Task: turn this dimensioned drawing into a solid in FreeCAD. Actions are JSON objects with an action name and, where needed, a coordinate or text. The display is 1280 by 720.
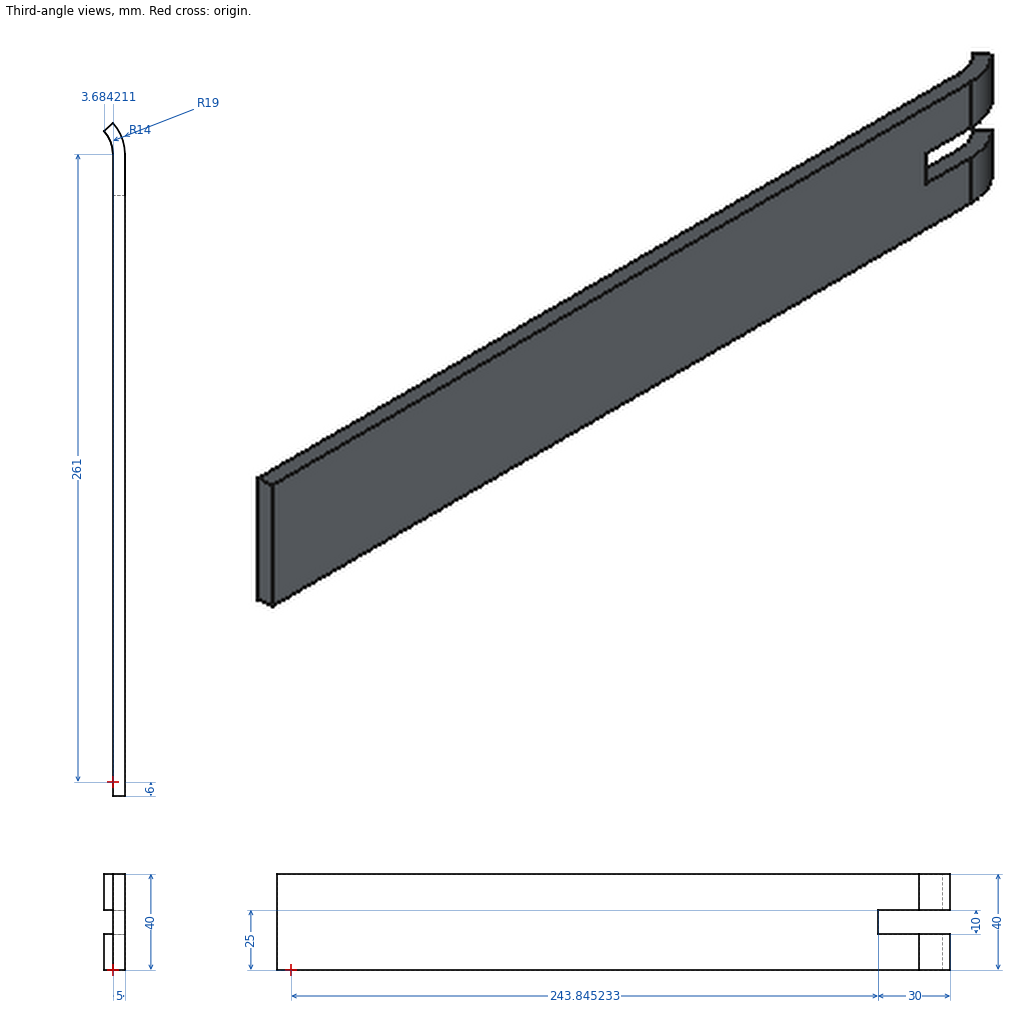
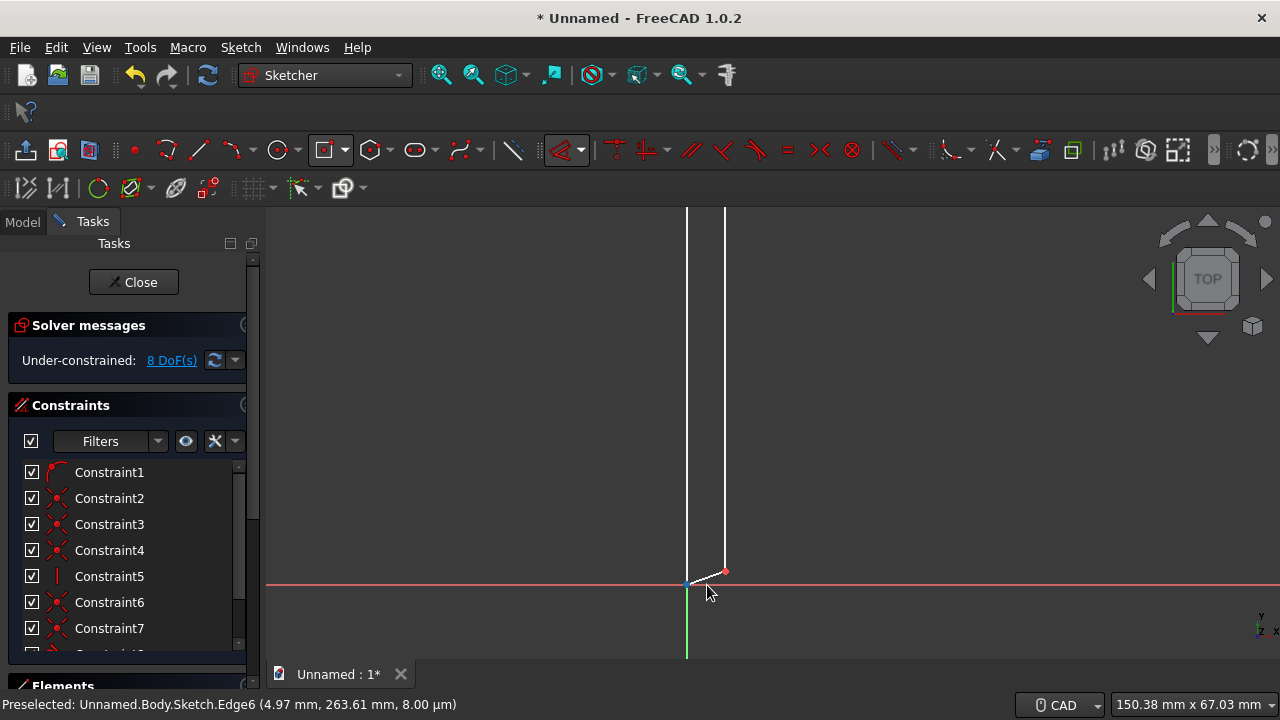
{"action": "left_click", "coordinate": [702, 579]}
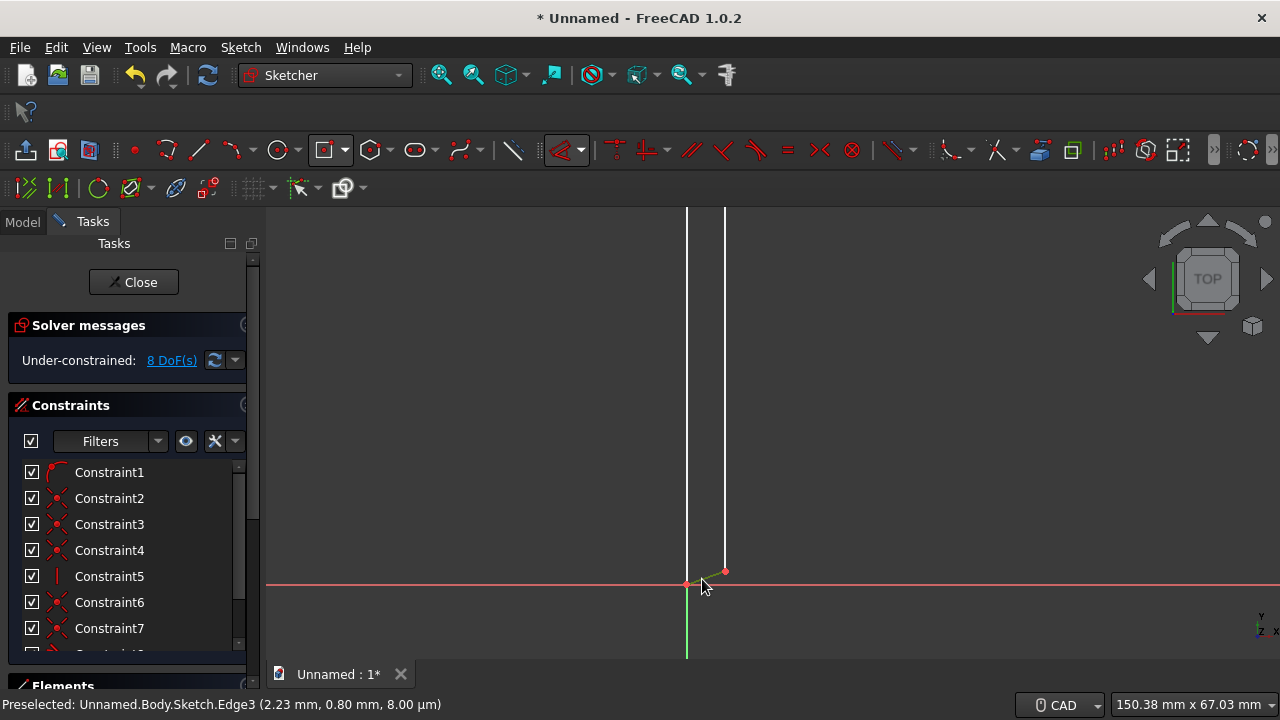
{"action": "key", "text": "h"}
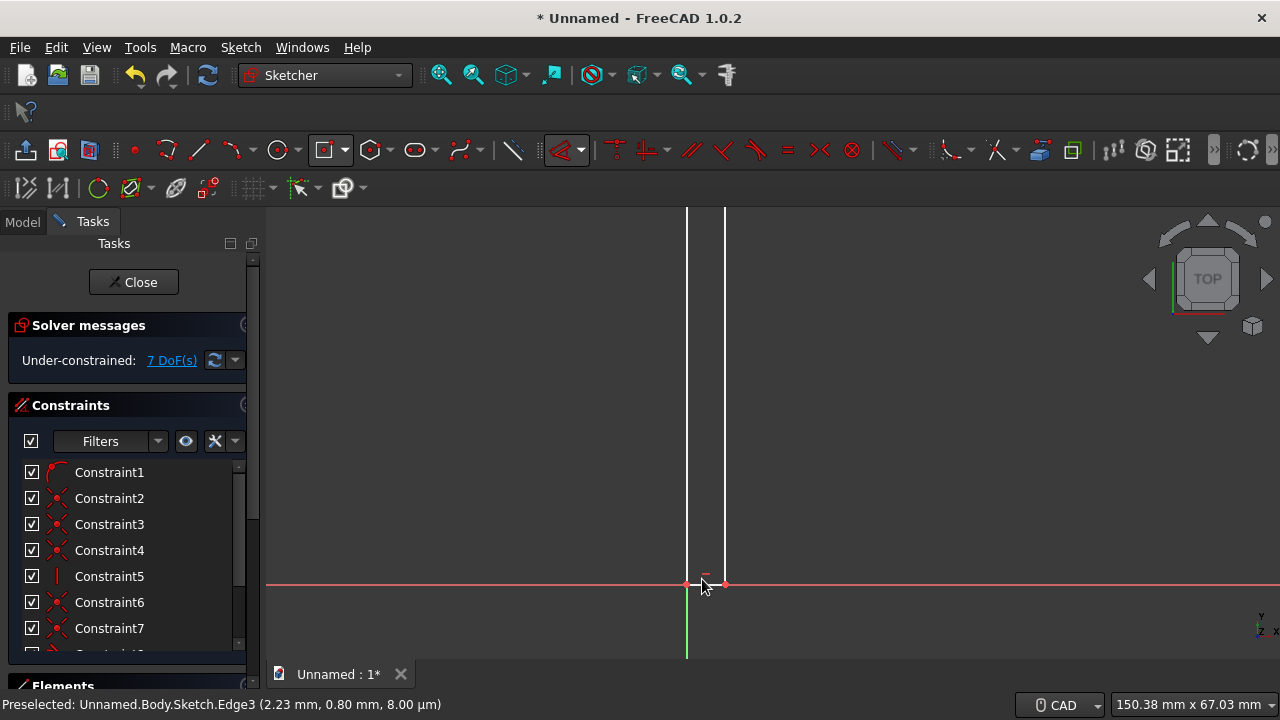
{"action": "scroll", "coordinate": [707, 586], "scroll_direction": "down", "scroll_amount": 9}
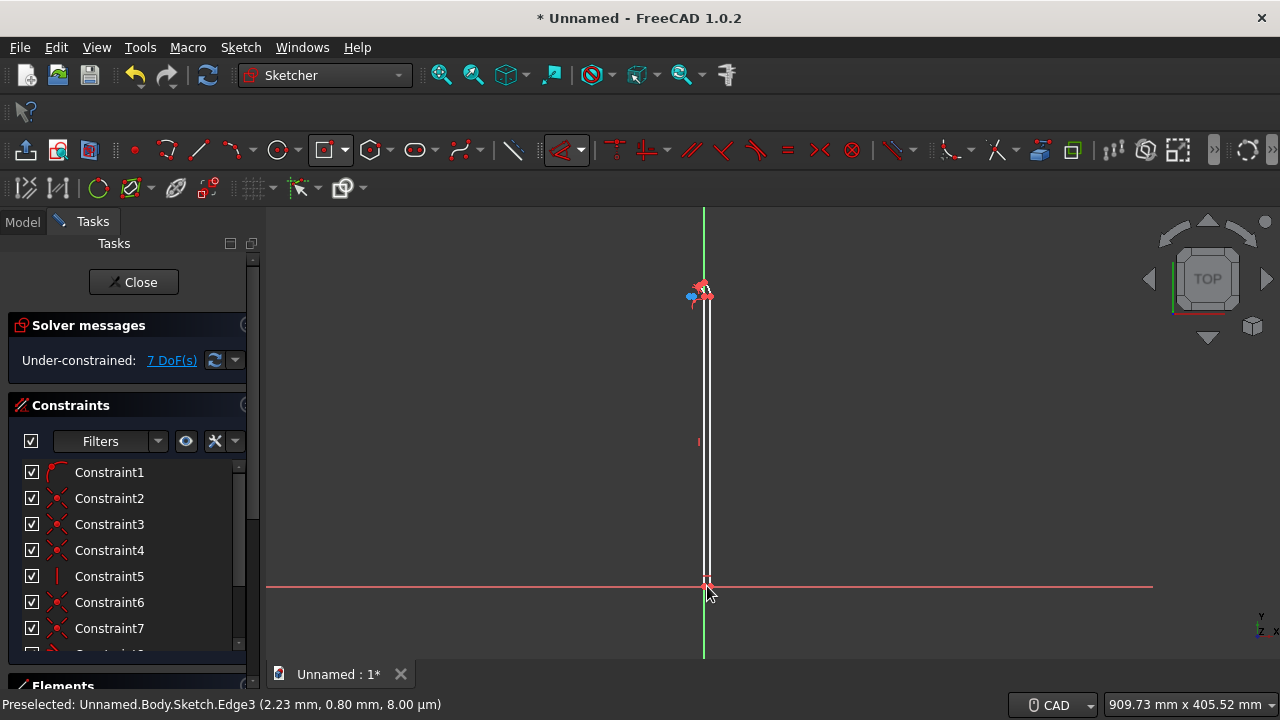
{"action": "scroll", "coordinate": [704, 293], "scroll_direction": "up", "scroll_amount": 7}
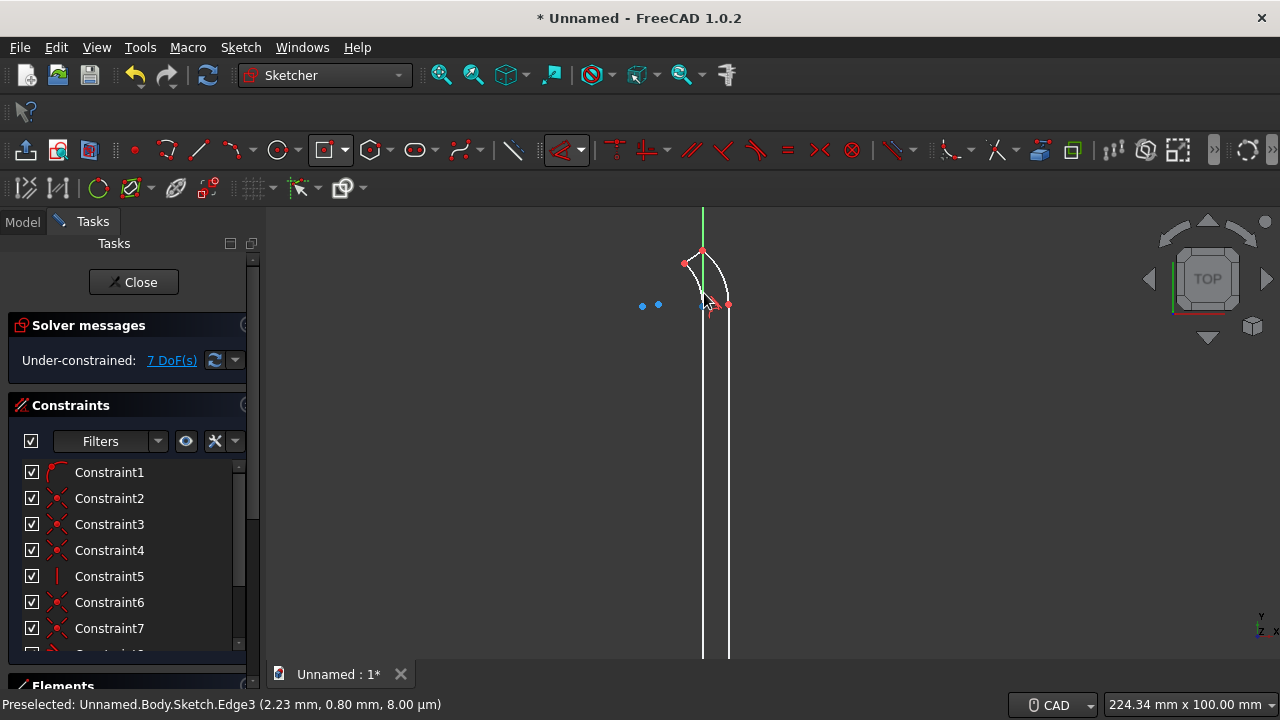
{"action": "left_click", "coordinate": [701, 292]}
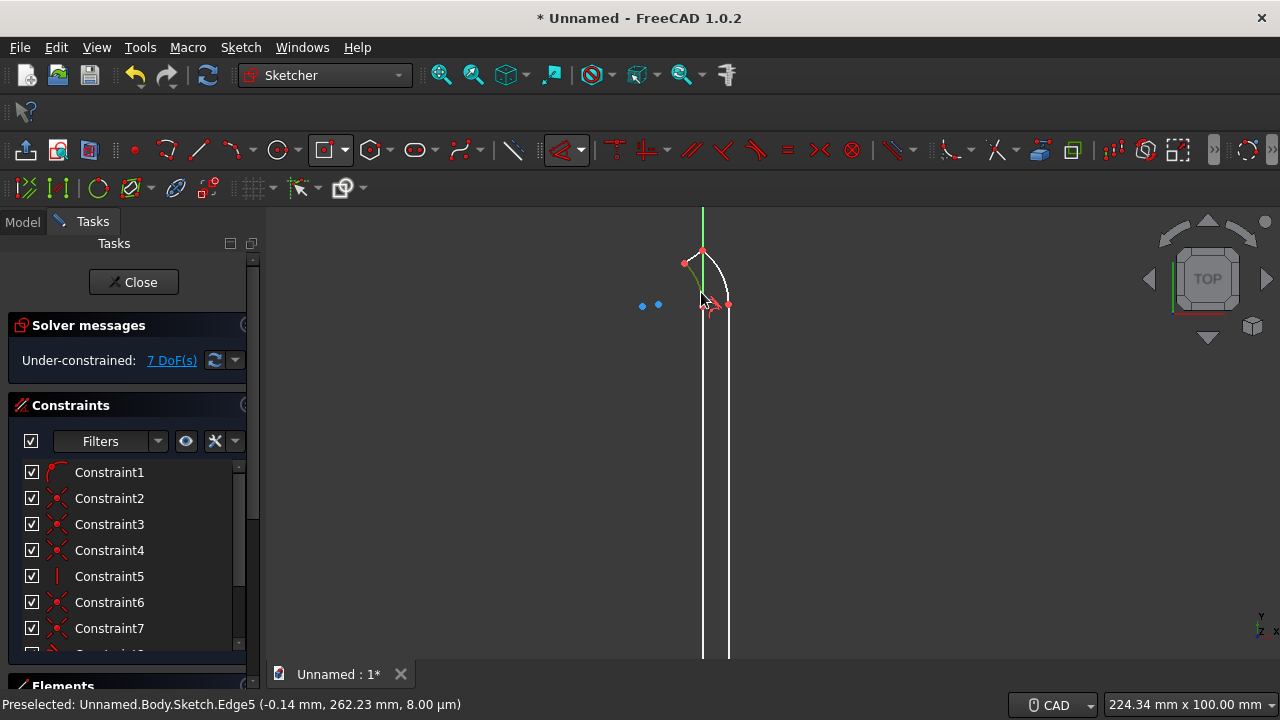
{"action": "left_click", "coordinate": [726, 286]}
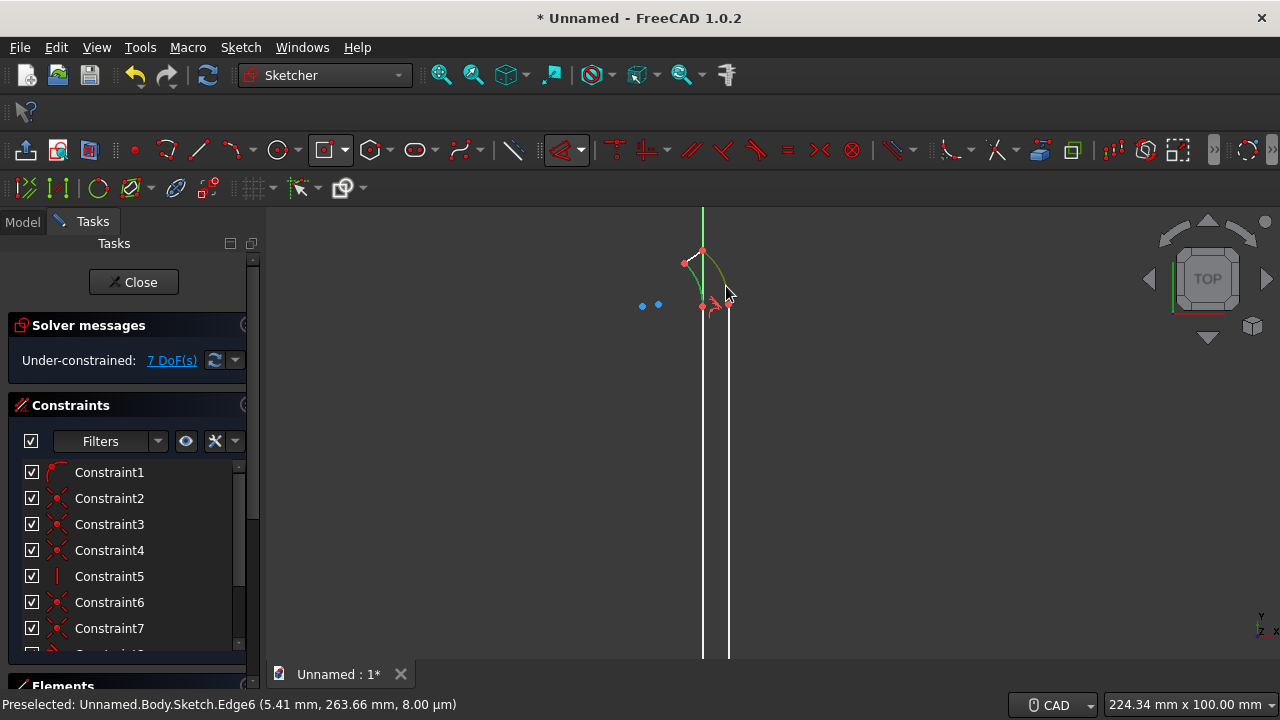
{"action": "left_click", "coordinate": [616, 150]}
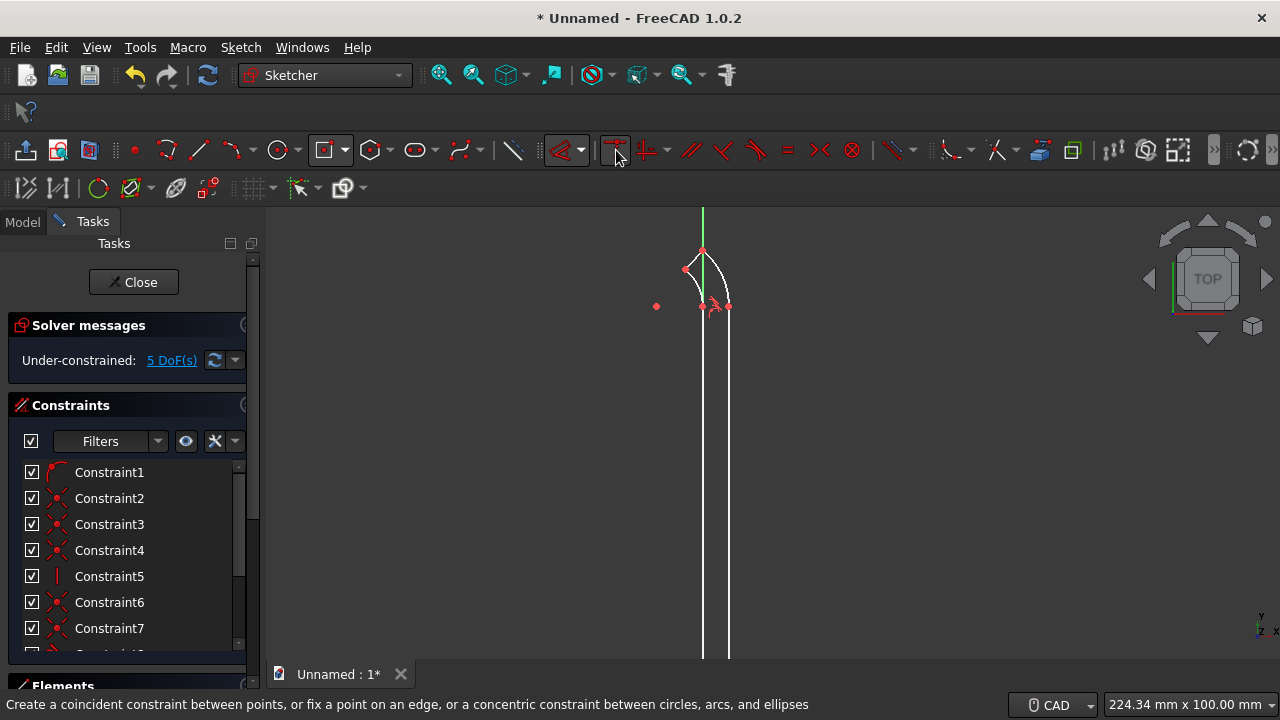
{"action": "left_click", "coordinate": [560, 150]}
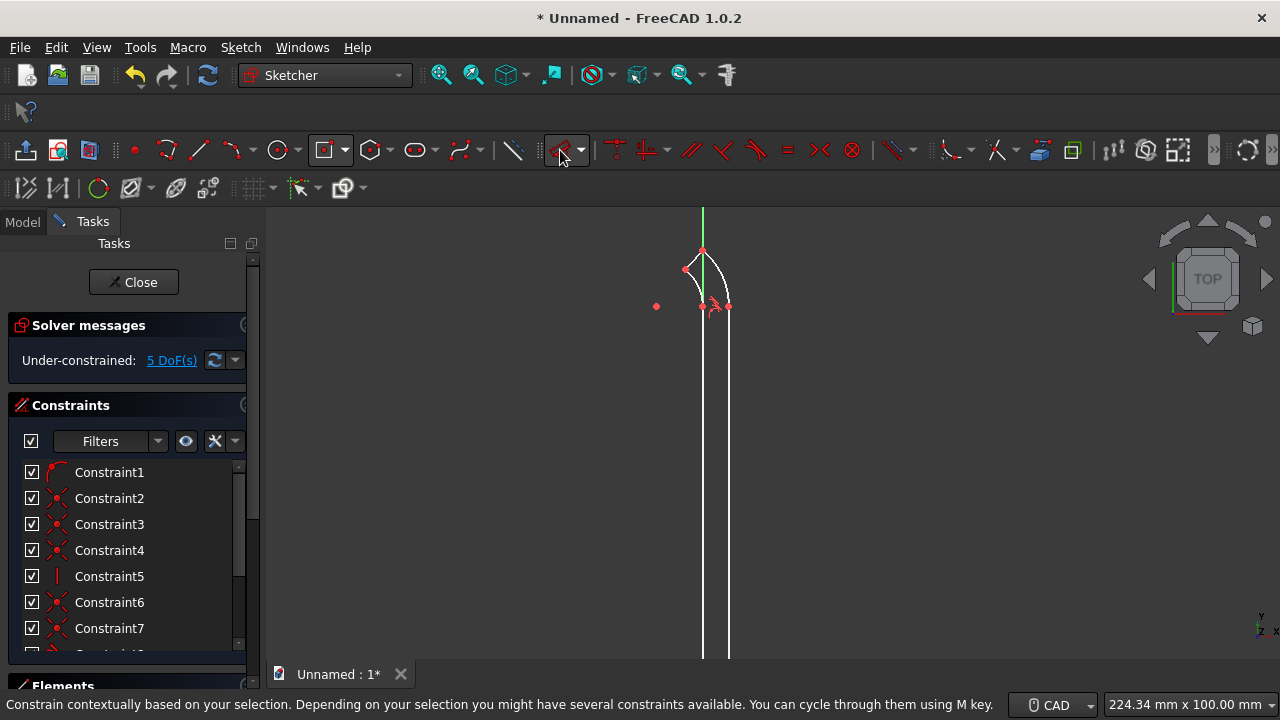
{"action": "left_click", "coordinate": [701, 294]}
{"action": "left_click", "coordinate": [677, 382]}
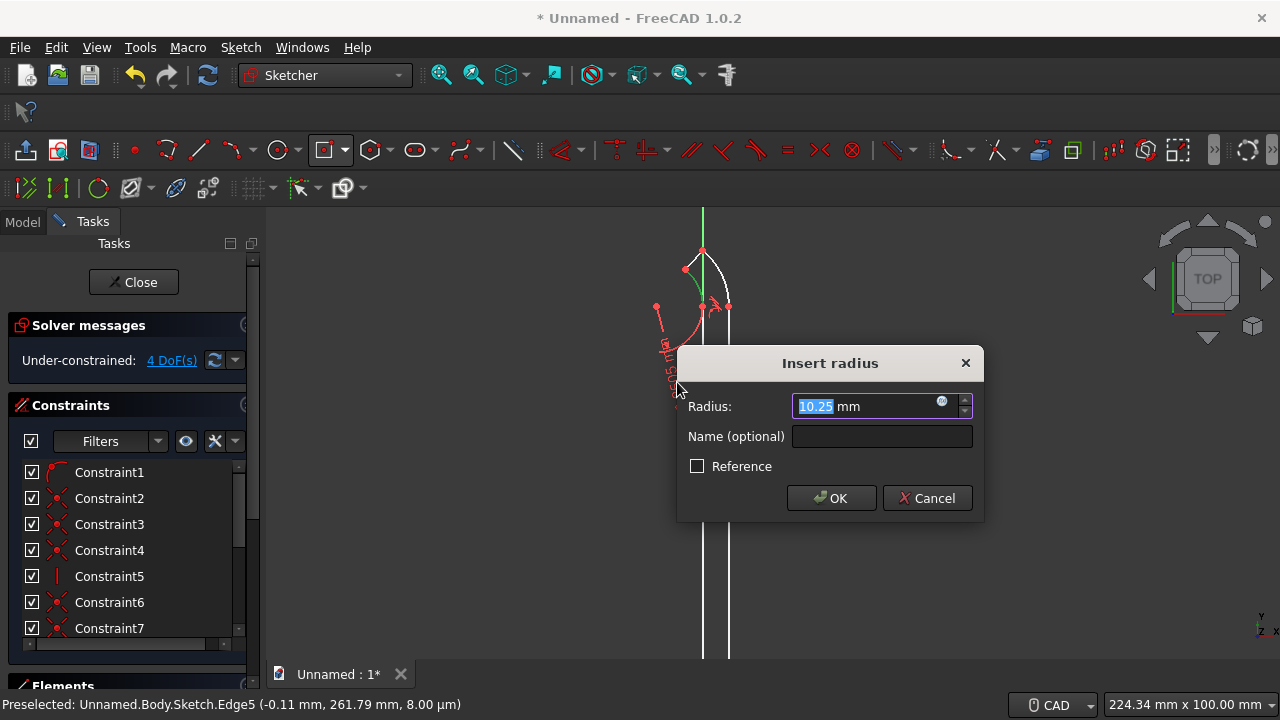
{"action": "type", "text": "14"}
{"action": "key", "text": "Return"}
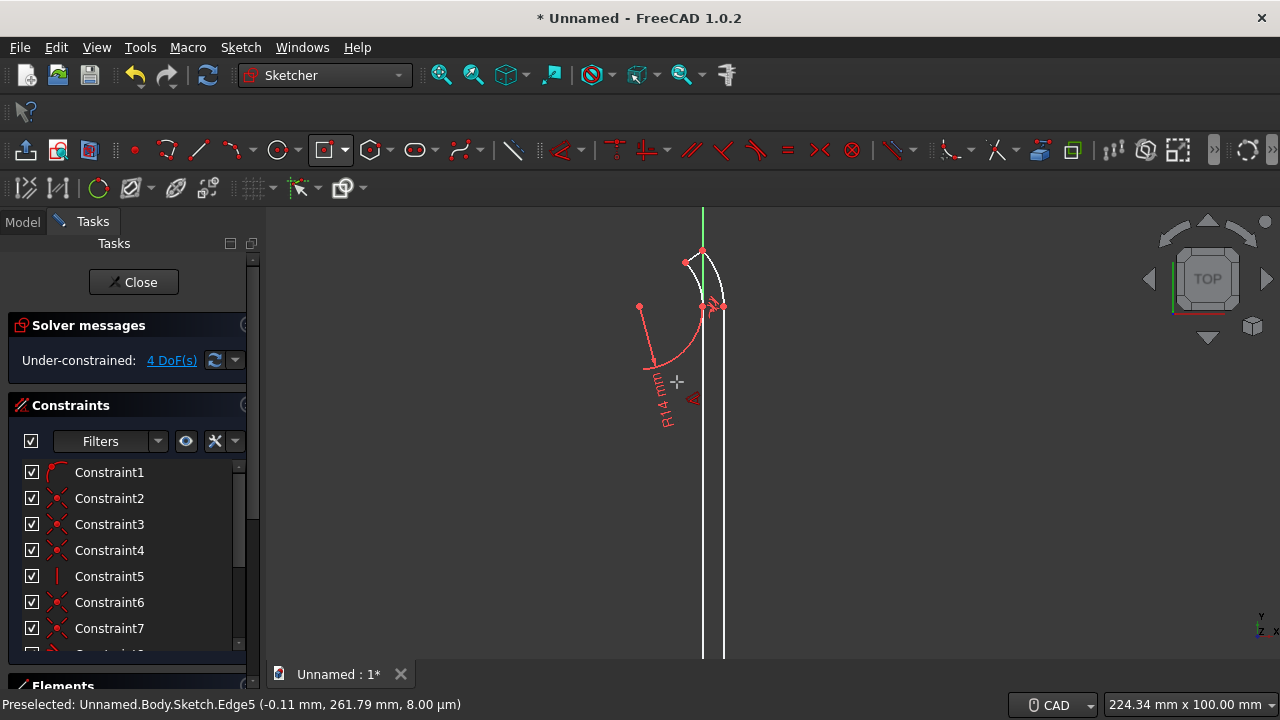
{"action": "left_click", "coordinate": [722, 288]}
{"action": "left_click", "coordinate": [753, 281]}